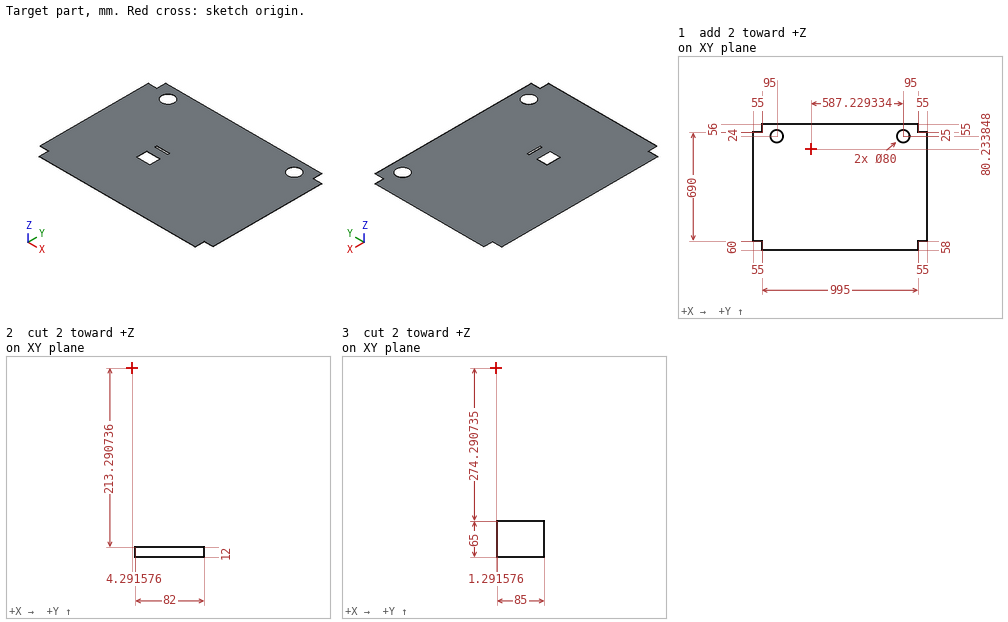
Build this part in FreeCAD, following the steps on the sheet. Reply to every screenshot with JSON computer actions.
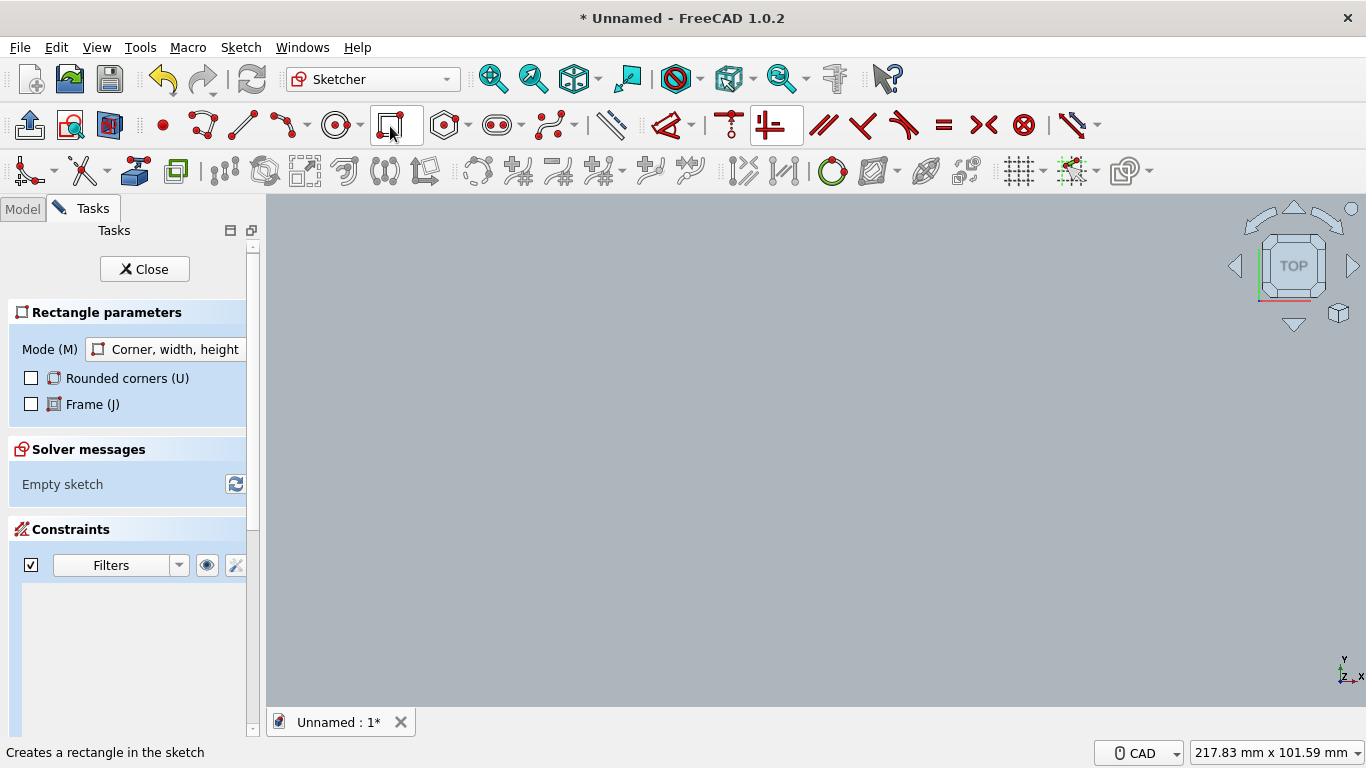
{"action": "scroll", "coordinate": [532, 285], "scroll_direction": "up", "scroll_amount": 5}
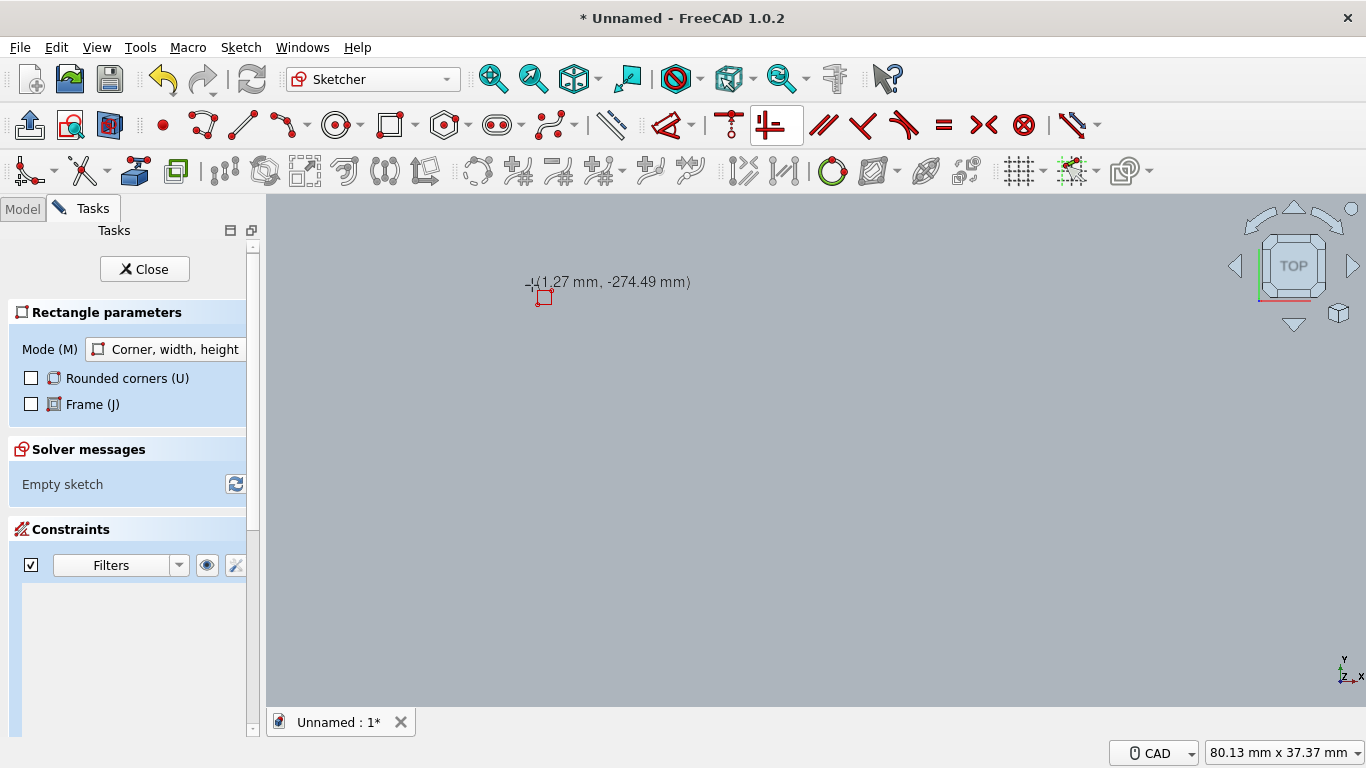
{"action": "left_click", "coordinate": [532, 285]}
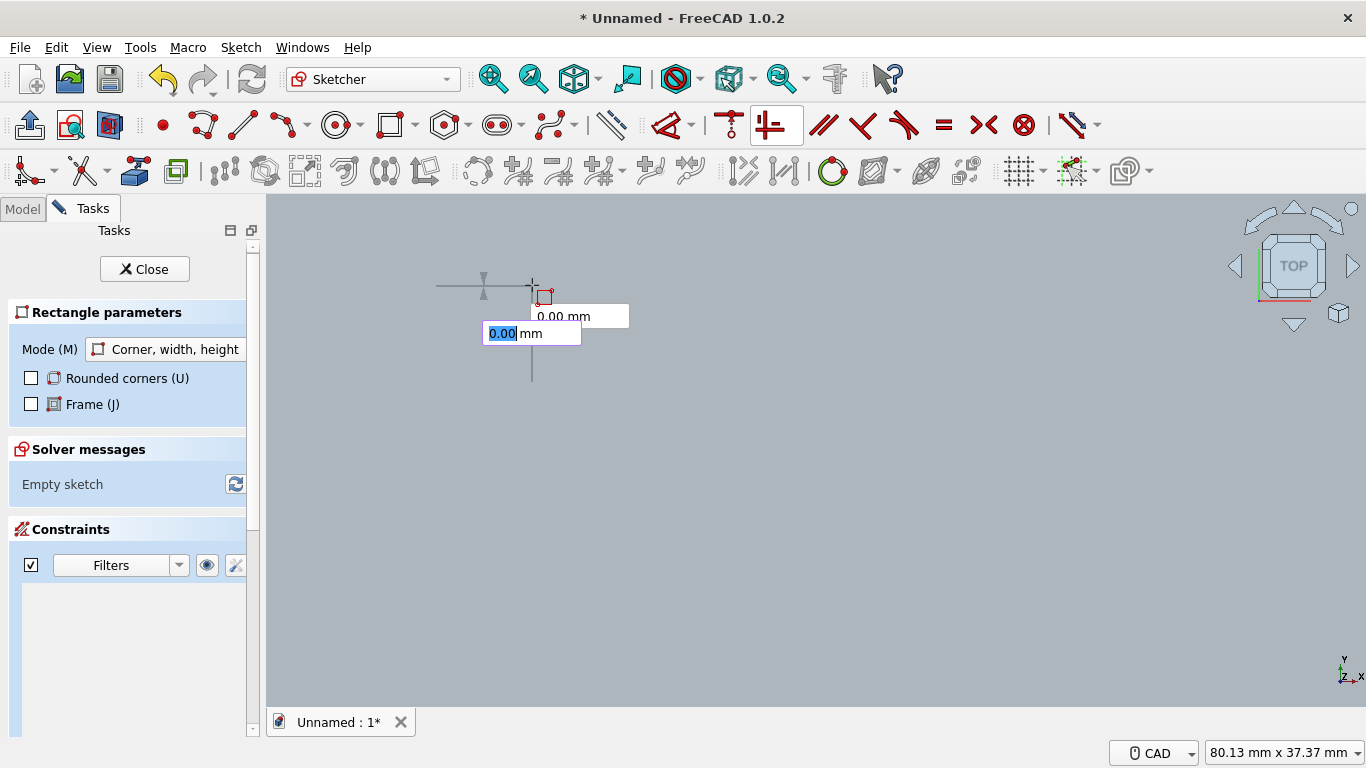
{"action": "scroll", "coordinate": [533, 287], "scroll_direction": "down", "scroll_amount": 5}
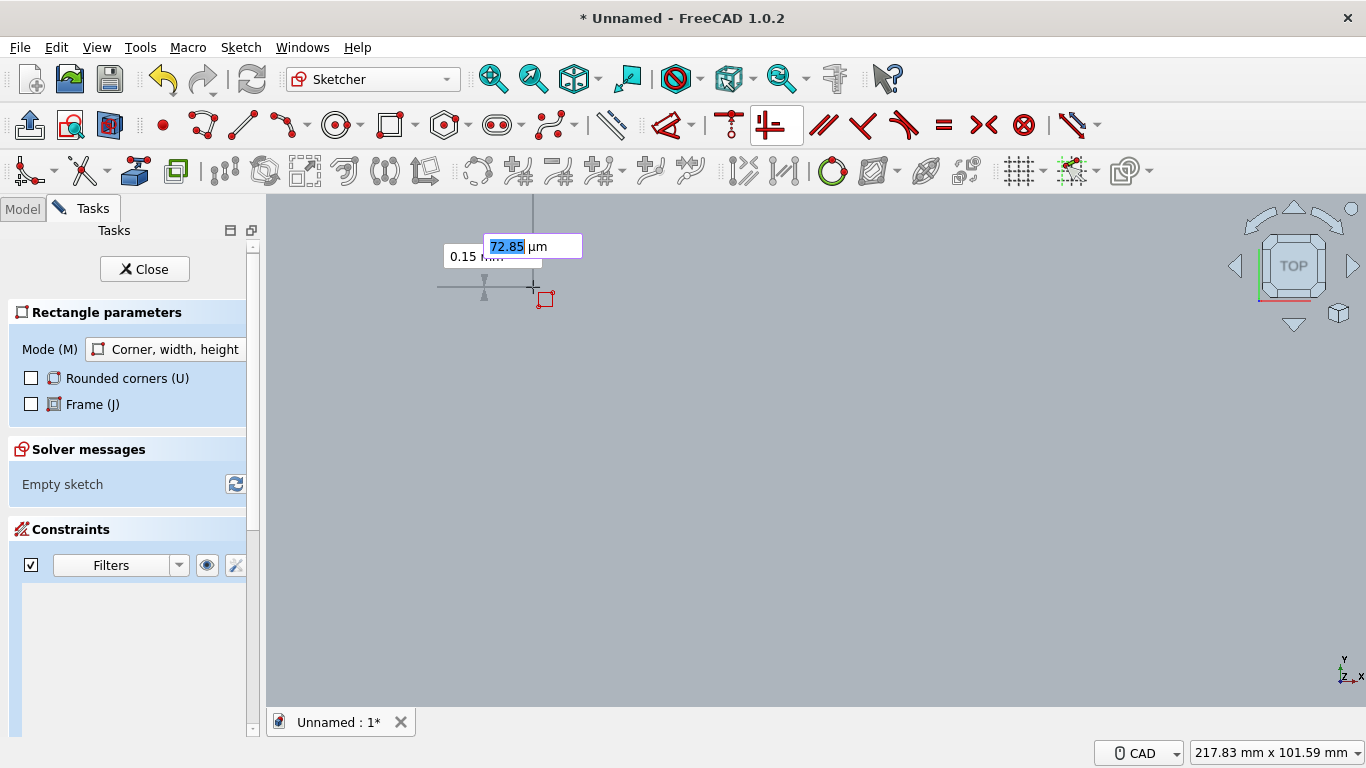
{"action": "left_click", "coordinate": [962, 615]}
{"action": "key", "text": "Escape"}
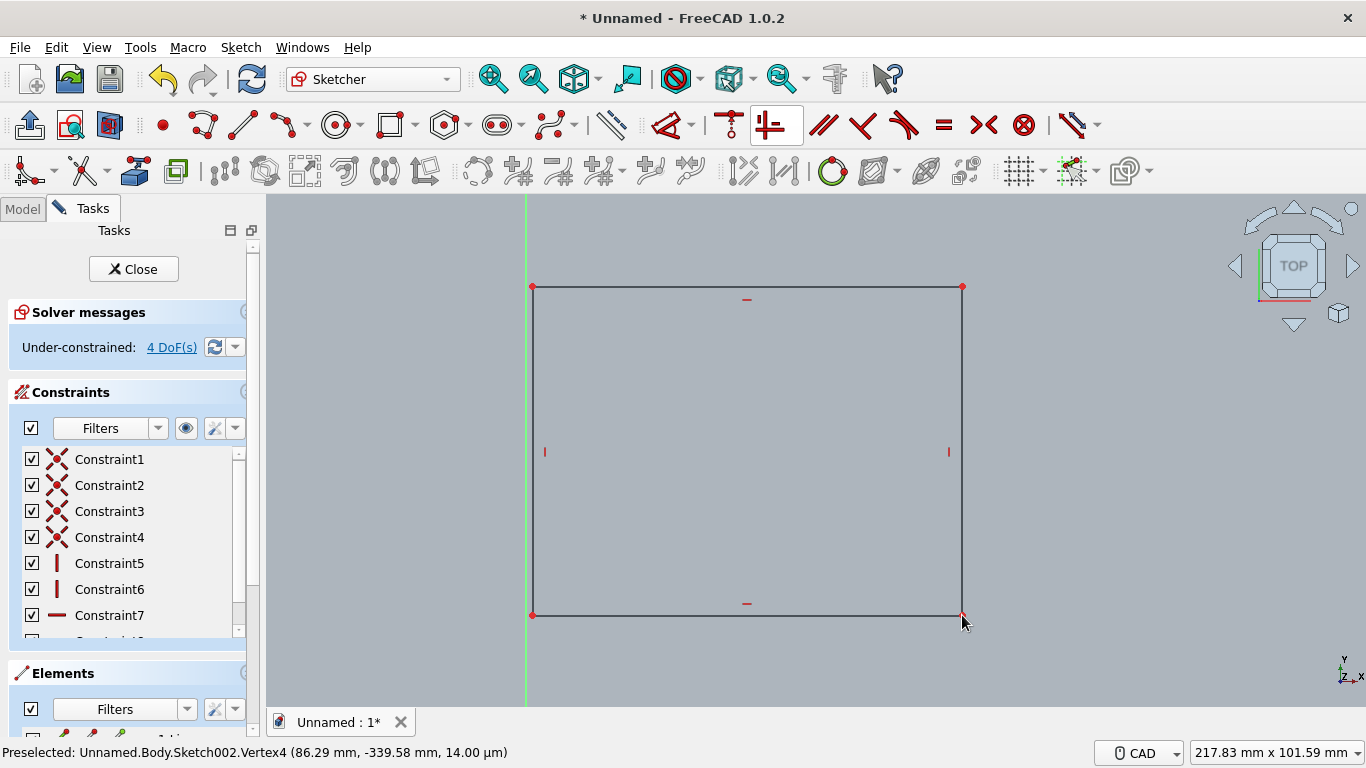
{"action": "left_click", "coordinate": [666, 126]}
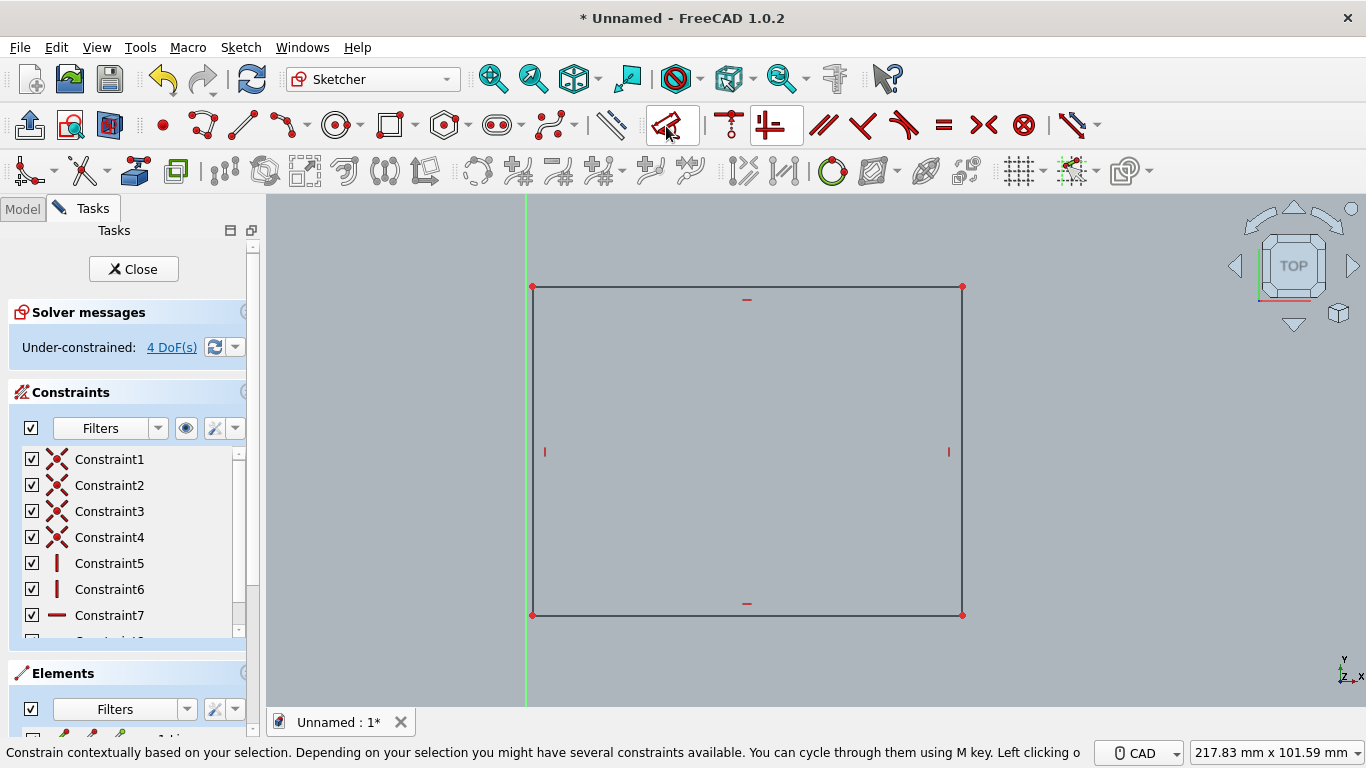
{"action": "scroll", "coordinate": [533, 386], "scroll_direction": "up", "scroll_amount": 4}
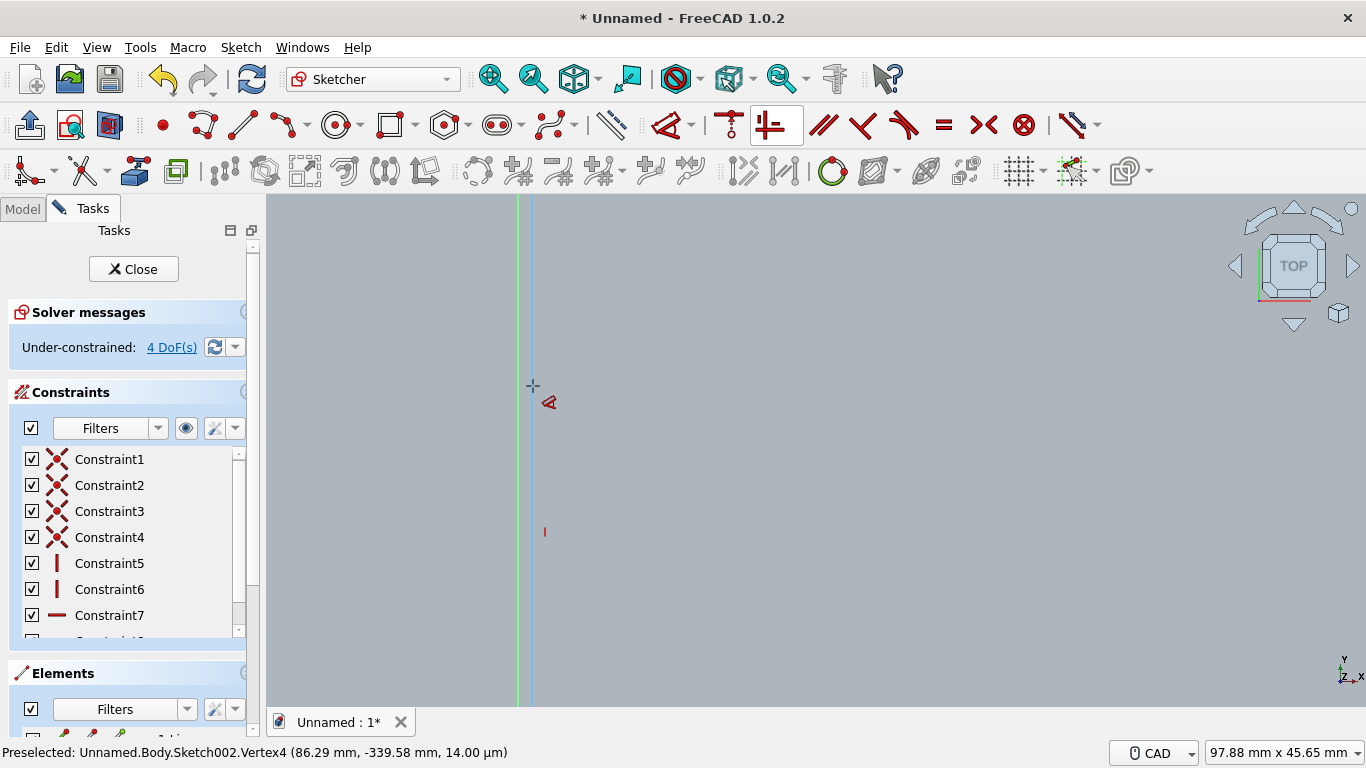
{"action": "left_click", "coordinate": [532, 384]}
{"action": "left_click", "coordinate": [498, 450]}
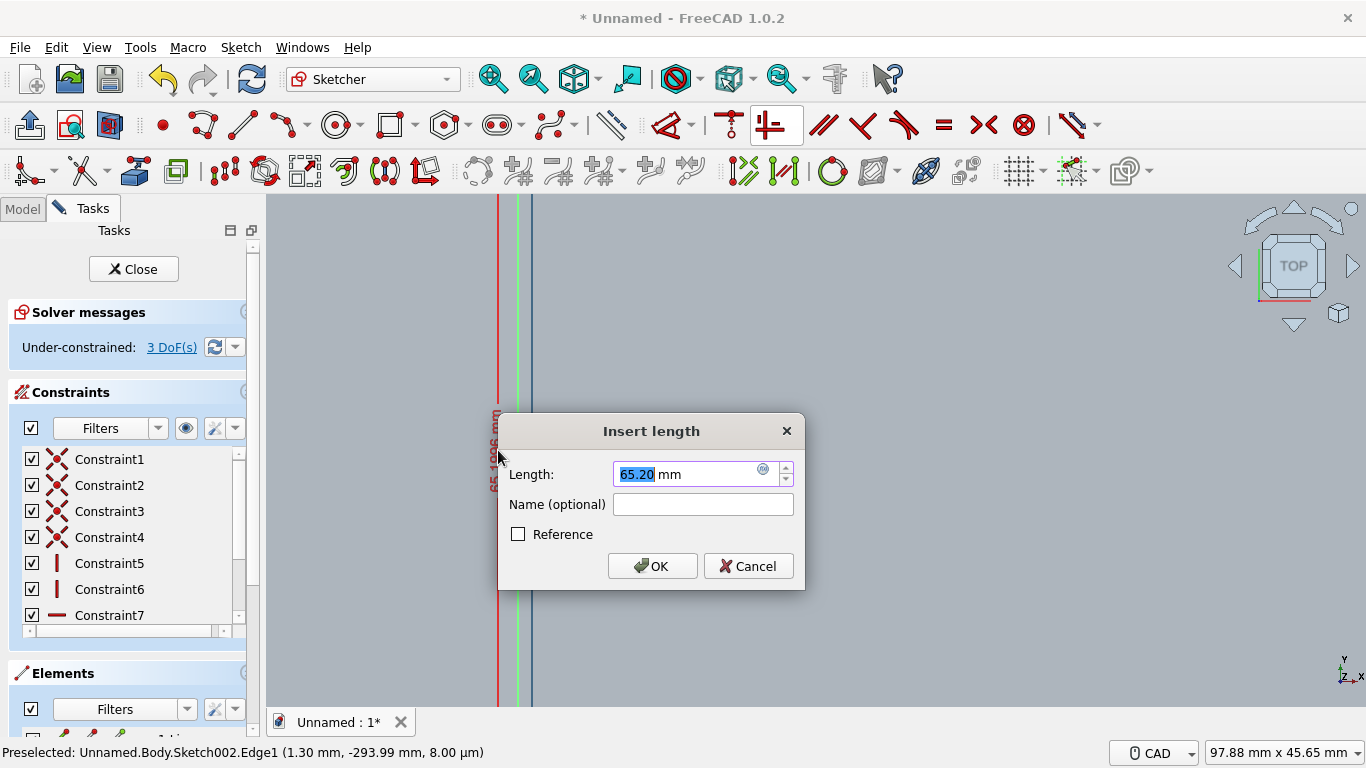
{"action": "type", "text": "65"}
{"action": "key", "text": "Return"}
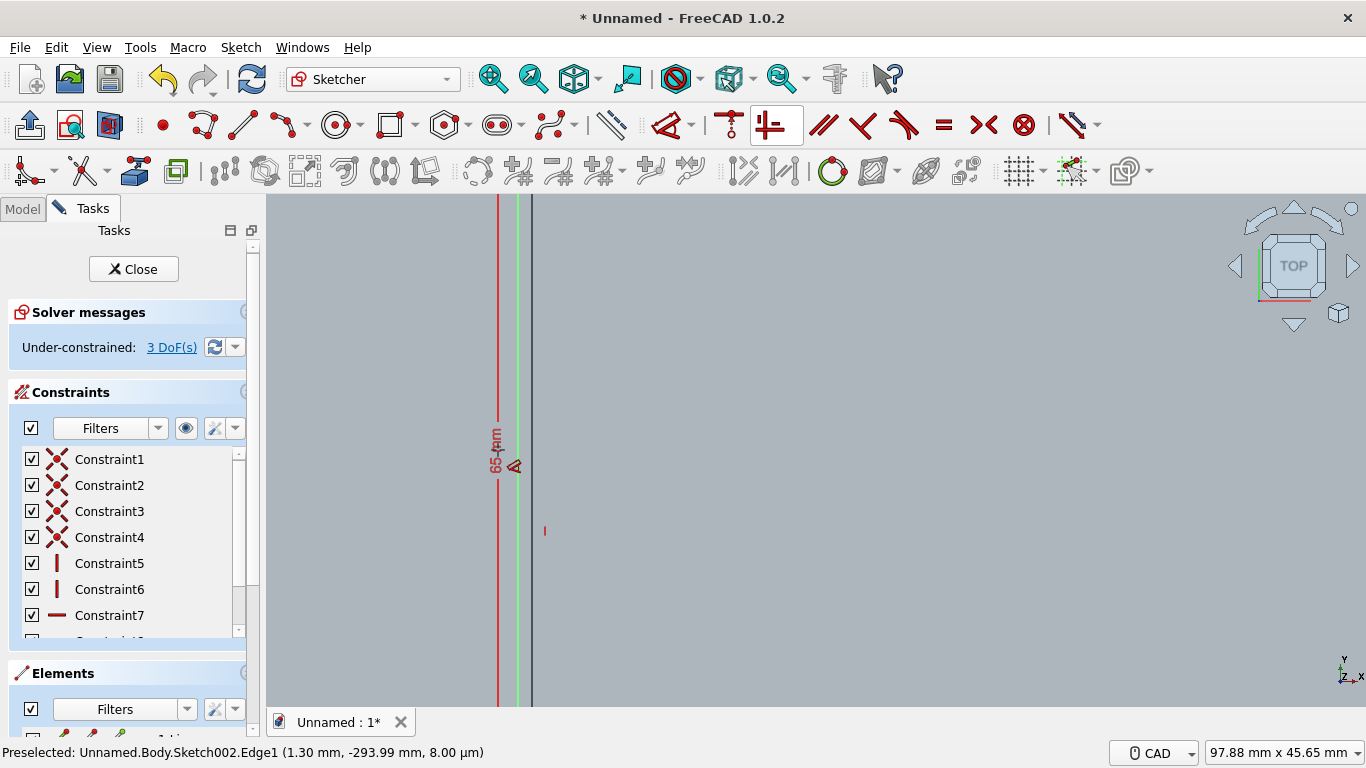
{"action": "scroll", "coordinate": [533, 387], "scroll_direction": "down", "scroll_amount": 4}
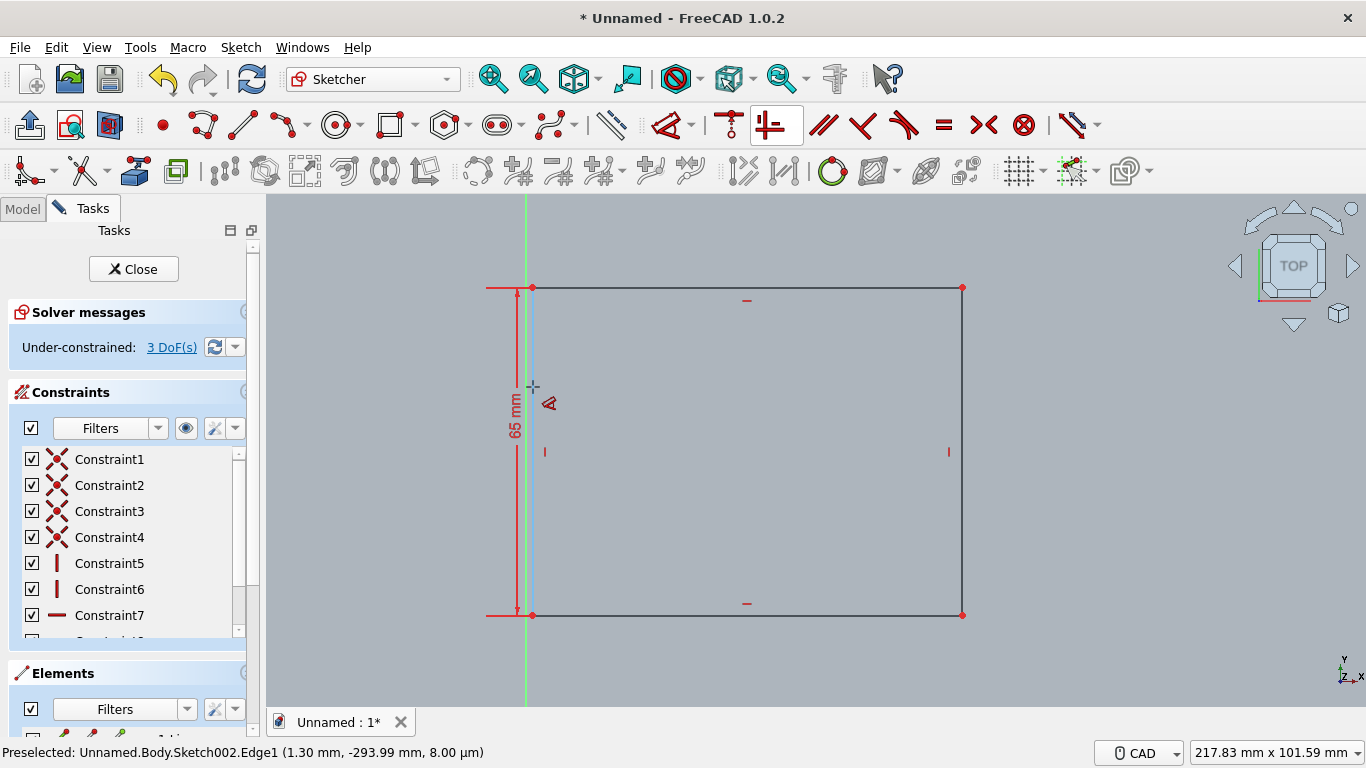
{"action": "left_click", "coordinate": [662, 616]}
{"action": "left_click", "coordinate": [747, 650]}